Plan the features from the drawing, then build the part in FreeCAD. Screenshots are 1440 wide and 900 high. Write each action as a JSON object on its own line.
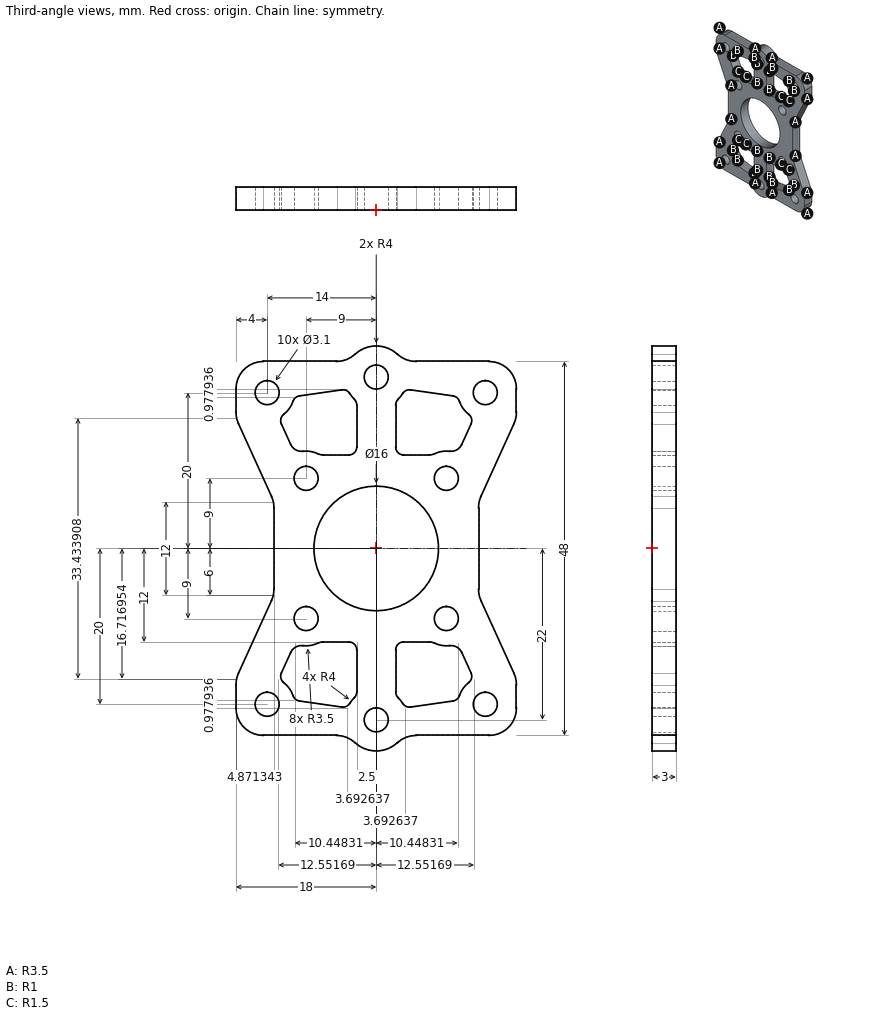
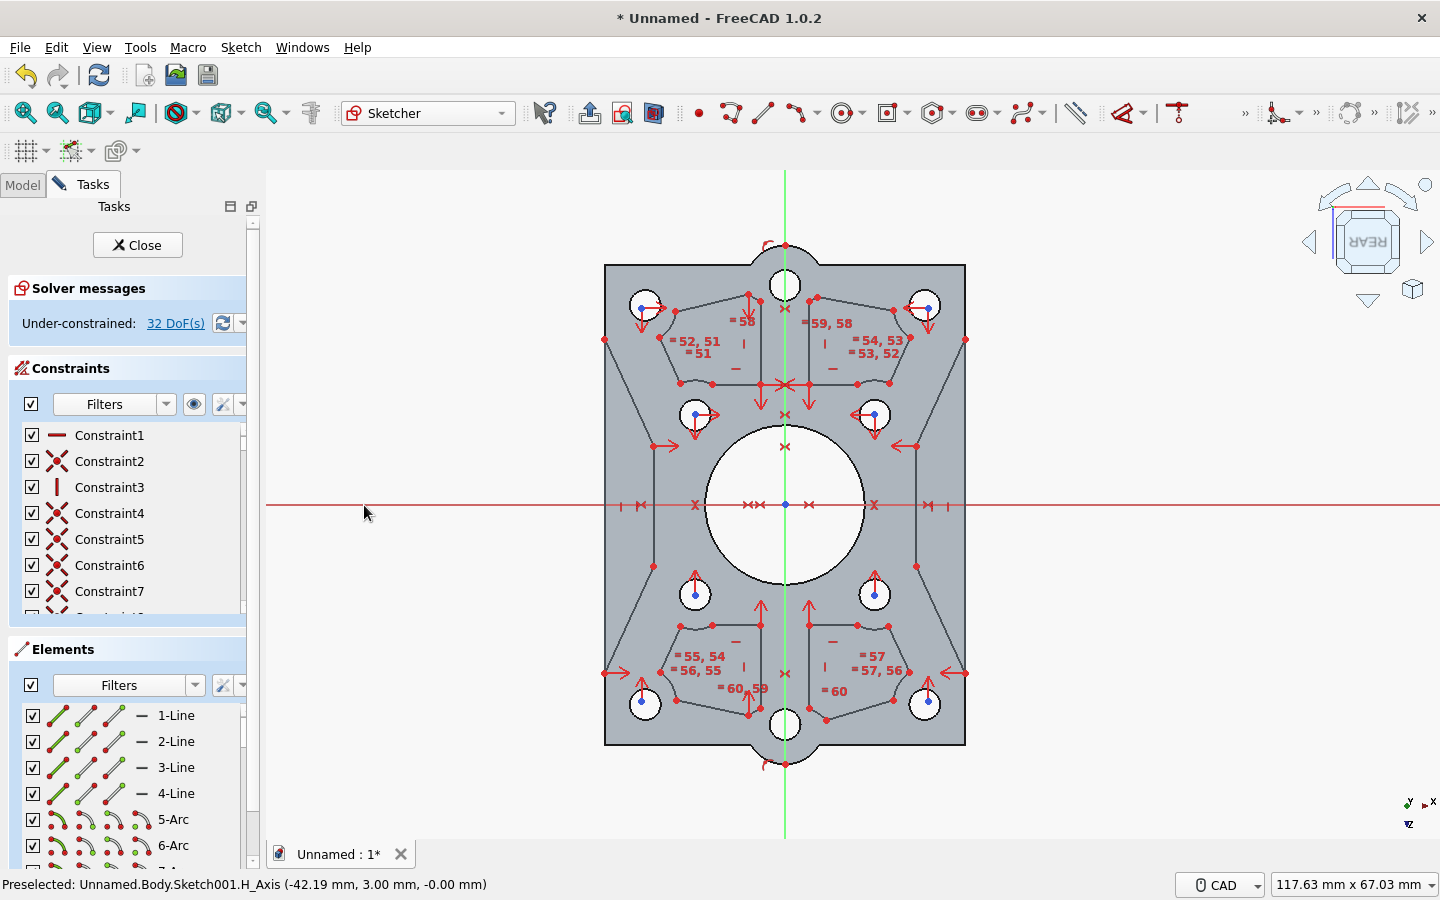
{"action": "left_click", "coordinate": [1122, 114]}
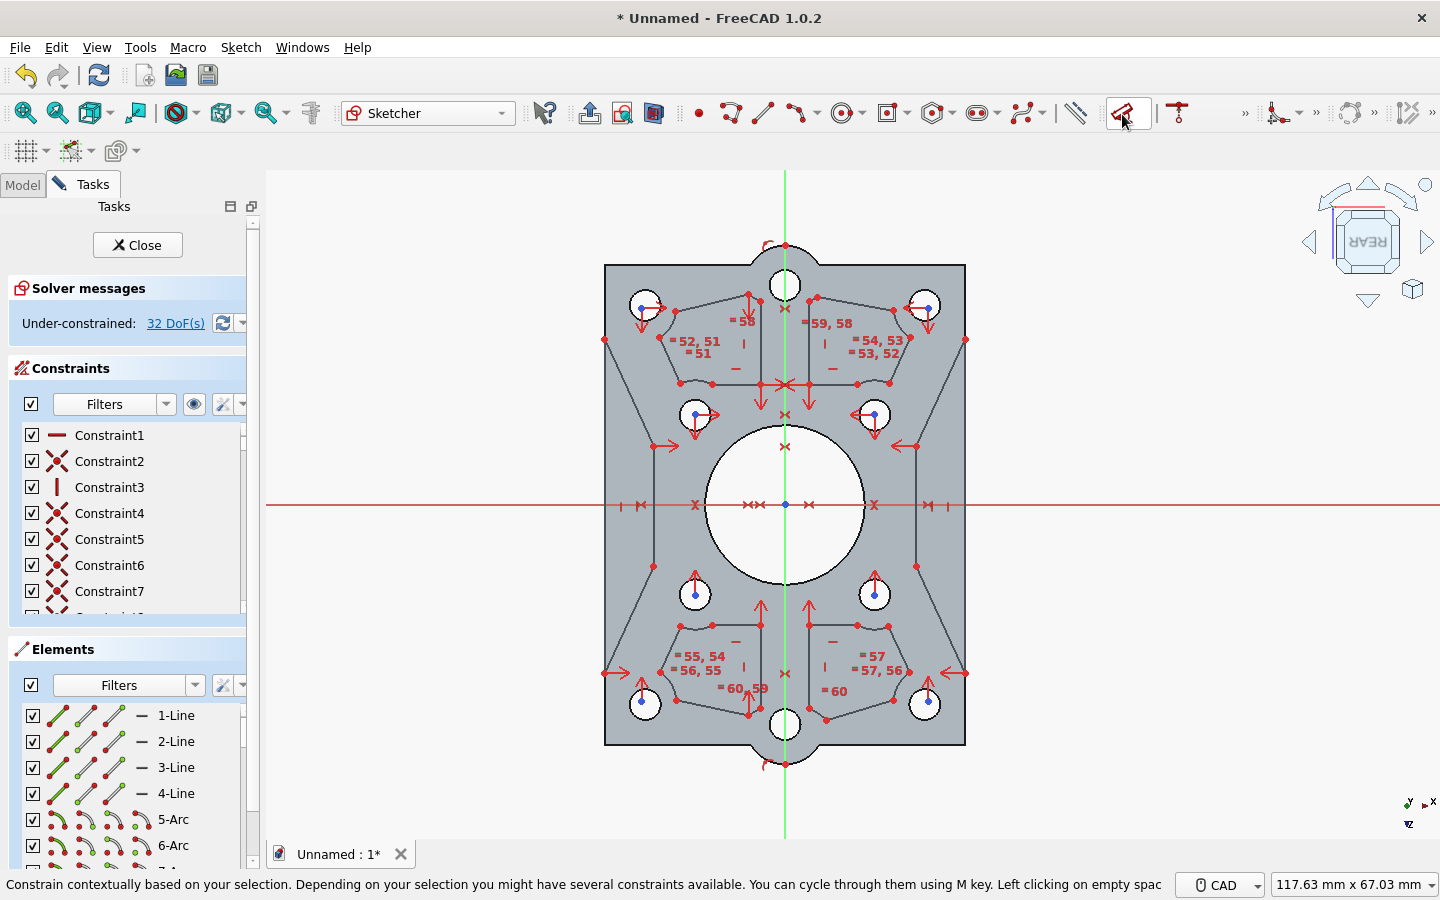
{"action": "scroll", "coordinate": [703, 381], "scroll_direction": "up", "scroll_amount": 2}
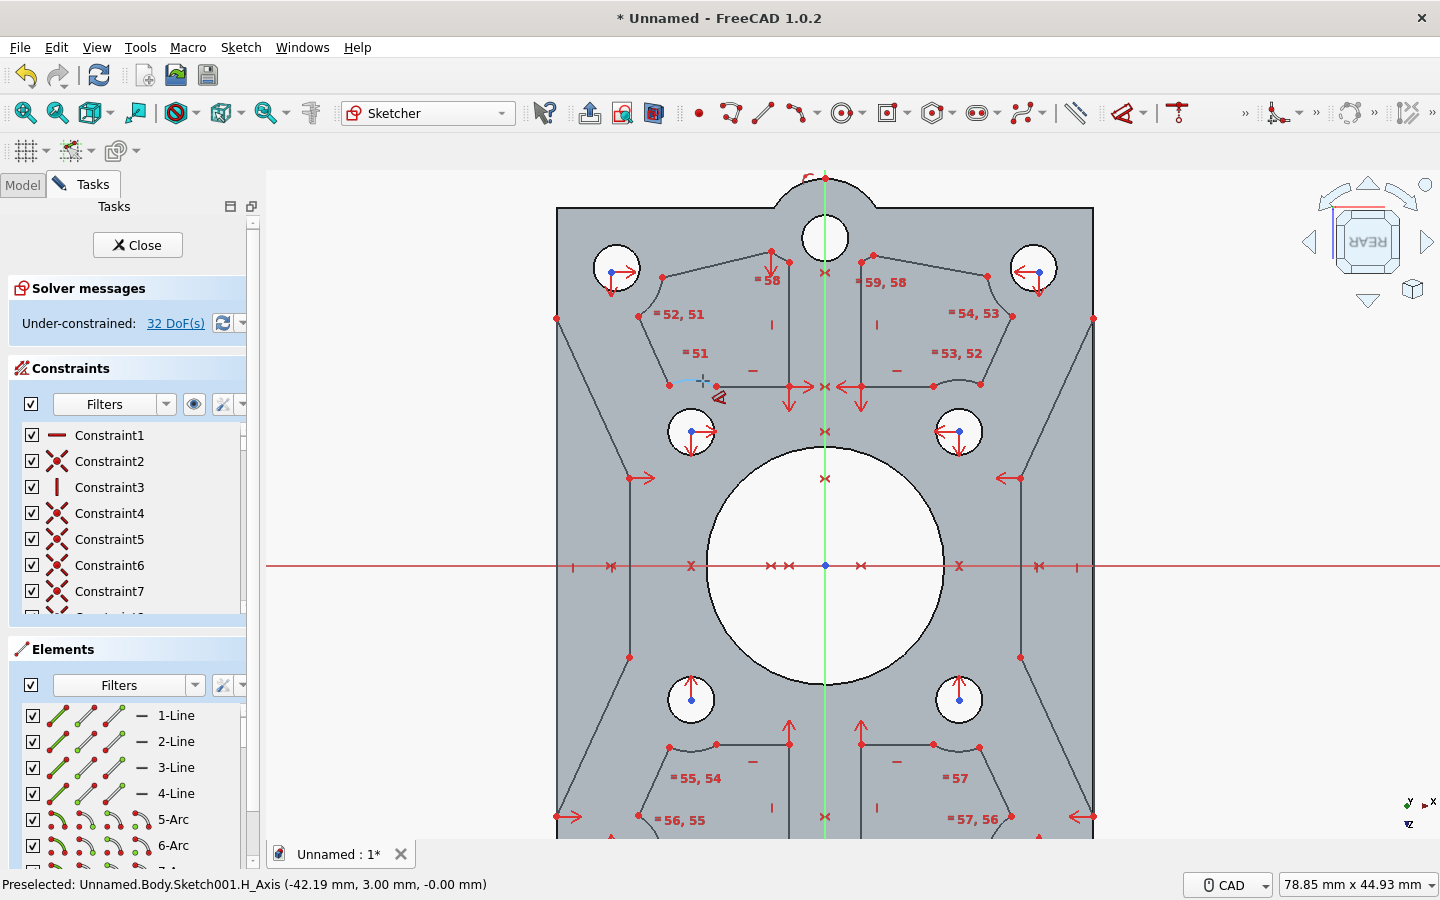
{"action": "left_click", "coordinate": [703, 381]}
{"action": "left_click", "coordinate": [710, 350]}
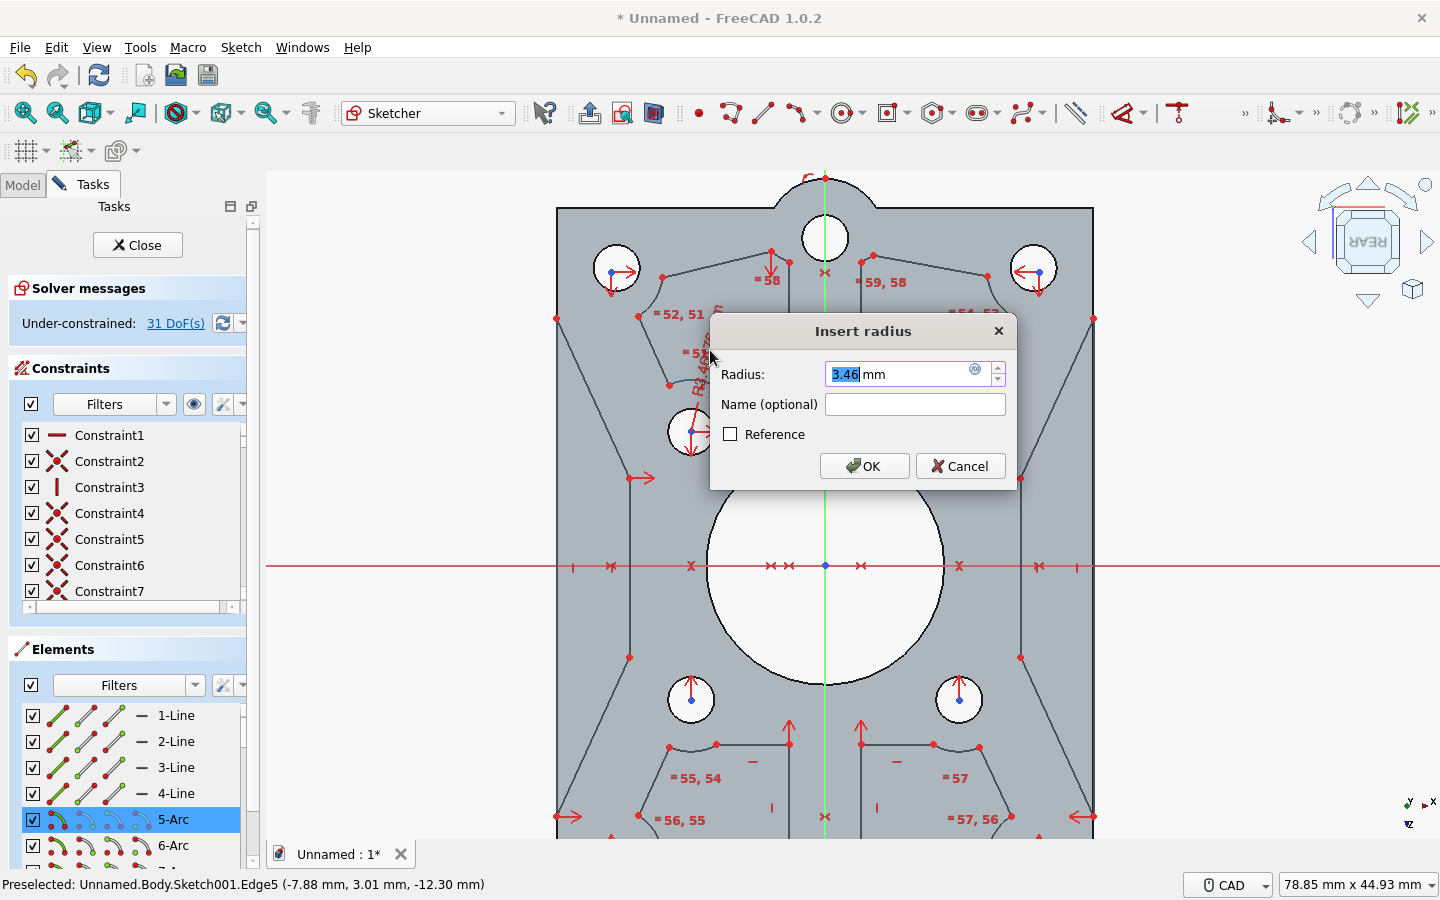
{"action": "type", "text": "3.5"}
{"action": "key", "text": "Return"}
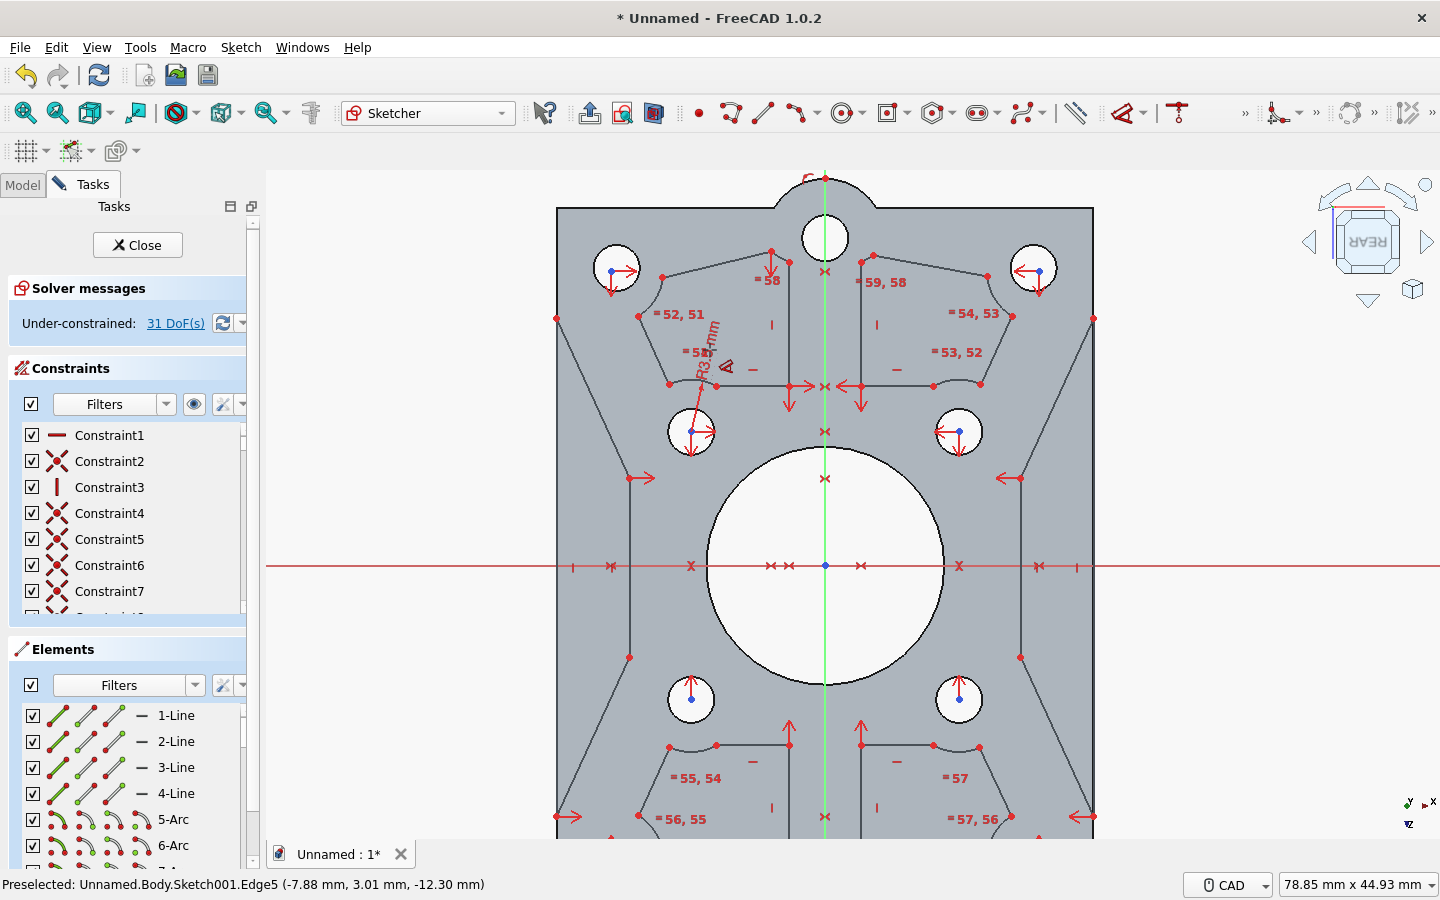
{"action": "scroll", "coordinate": [780, 257], "scroll_direction": "up", "scroll_amount": 2}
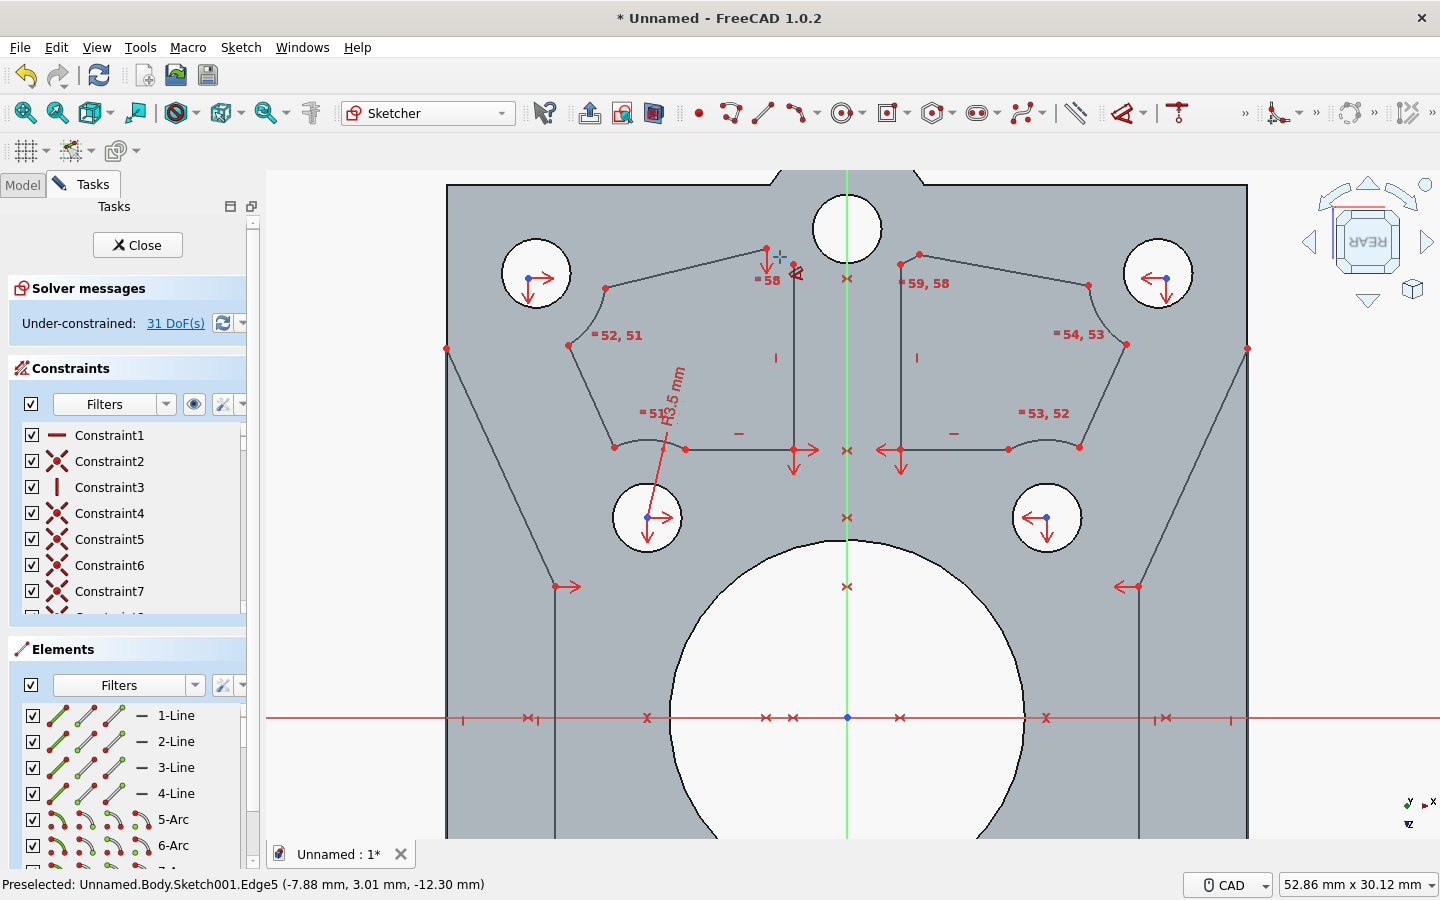
{"action": "left_click", "coordinate": [780, 257]}
{"action": "left_click", "coordinate": [764, 285]}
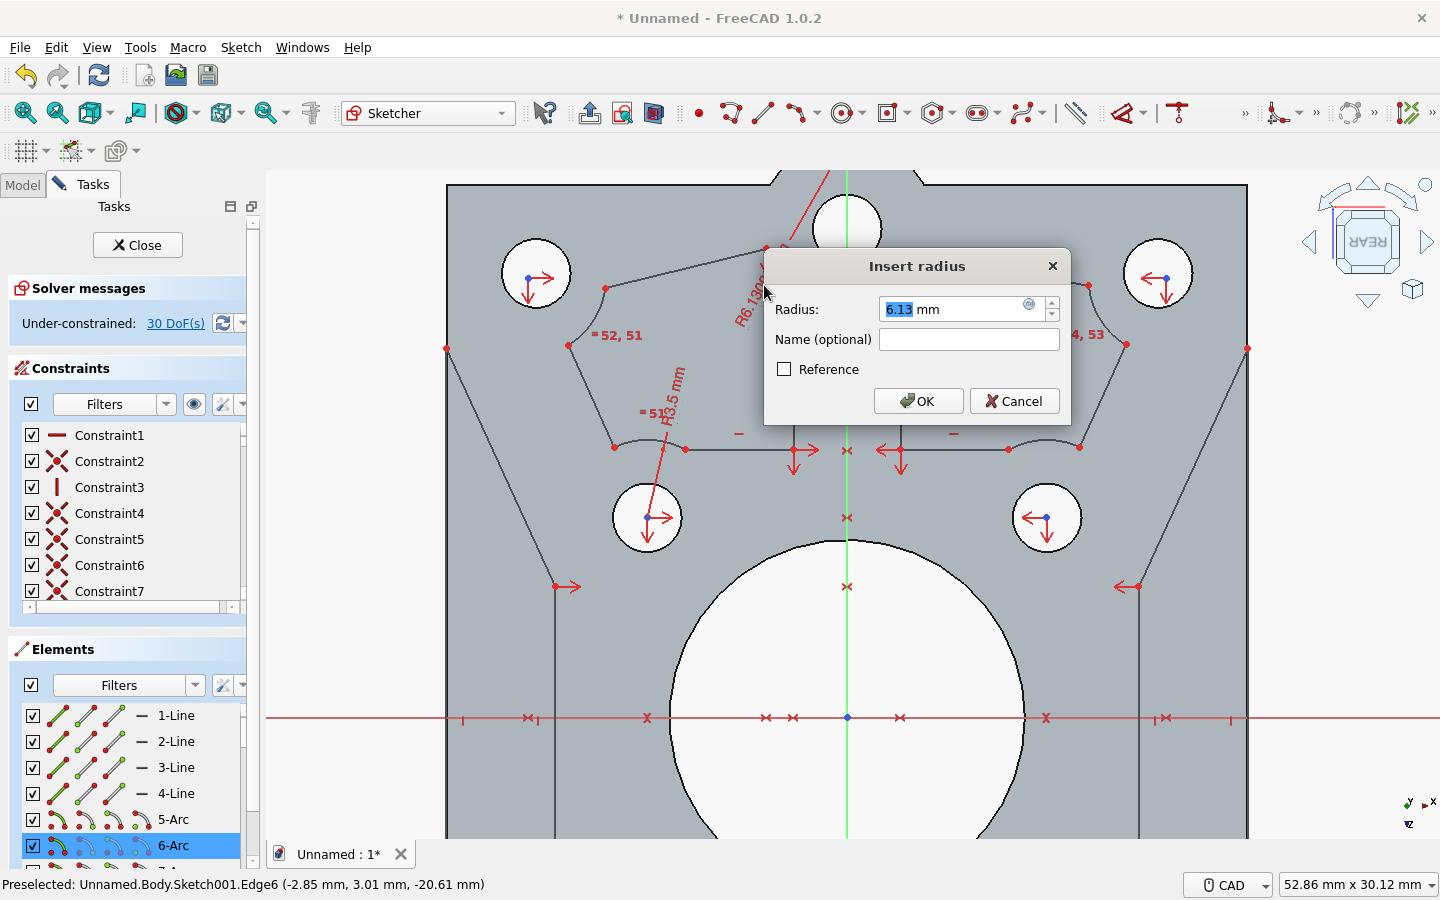
{"action": "type", "text": "4"}
{"action": "key", "text": "Return"}